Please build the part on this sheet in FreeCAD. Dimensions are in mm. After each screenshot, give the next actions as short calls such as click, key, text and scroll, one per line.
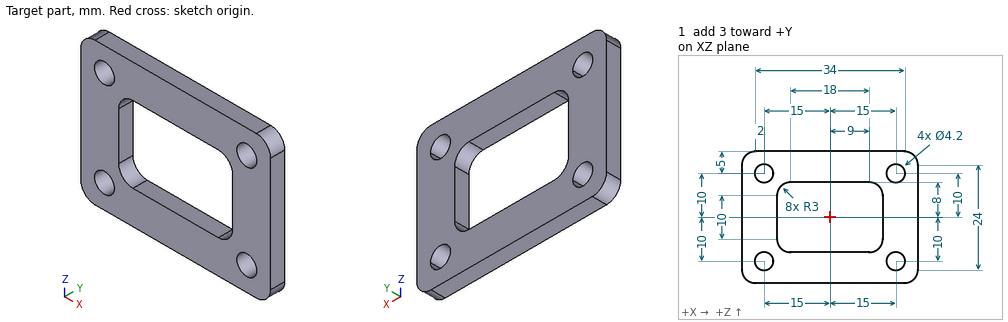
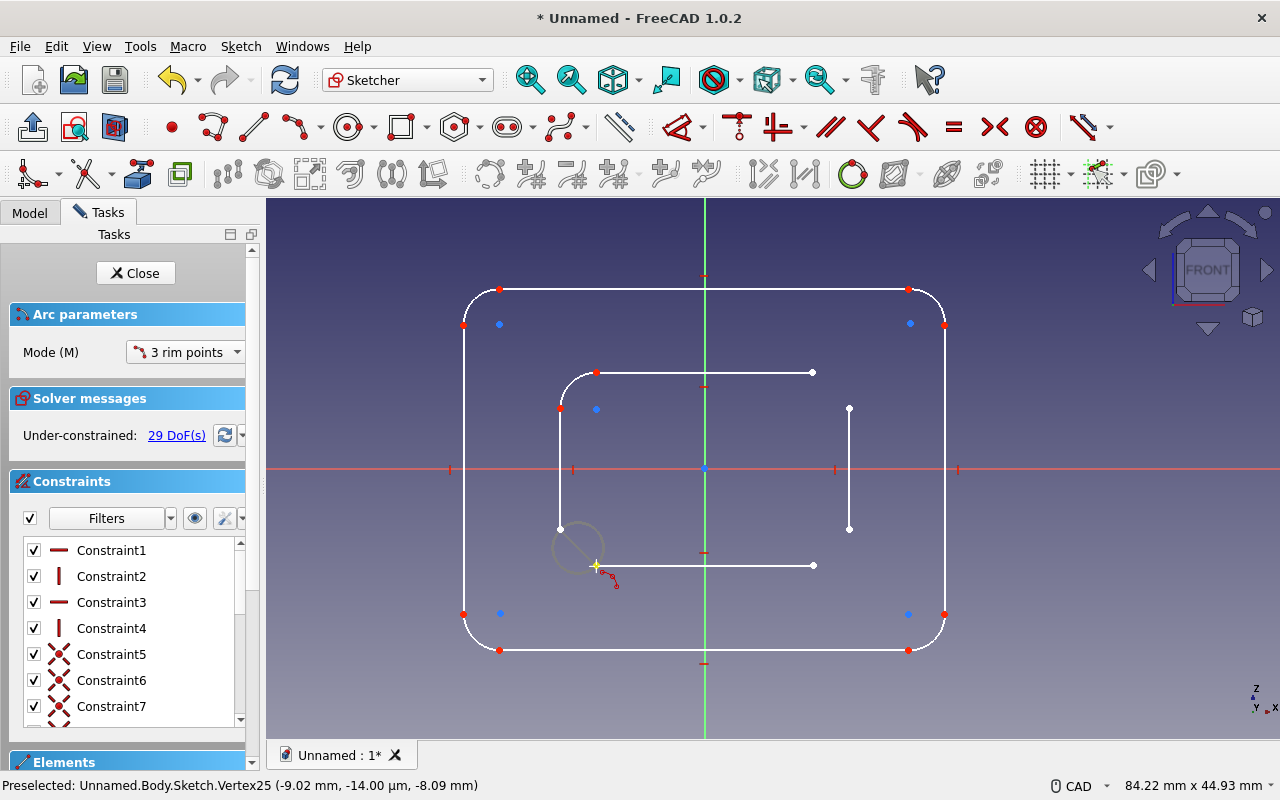
scroll(571, 554, up, 3)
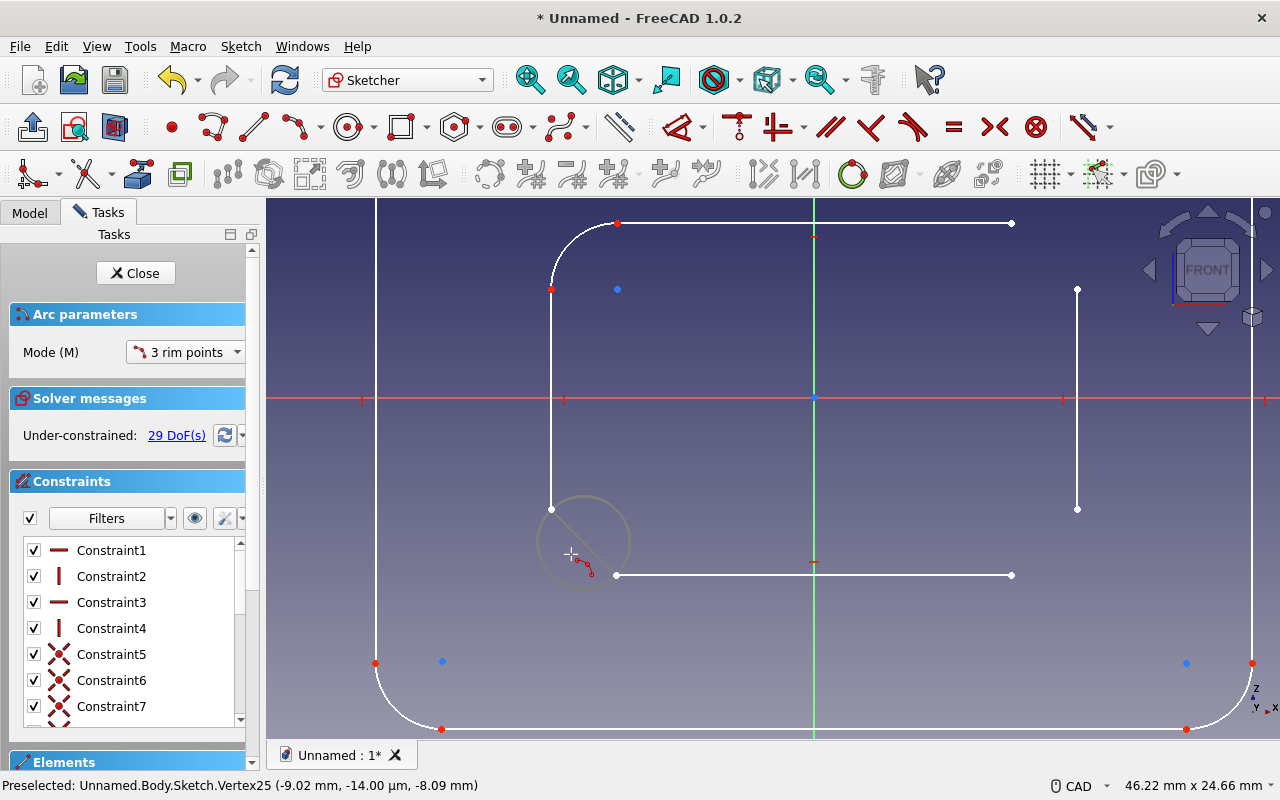
click(570, 554)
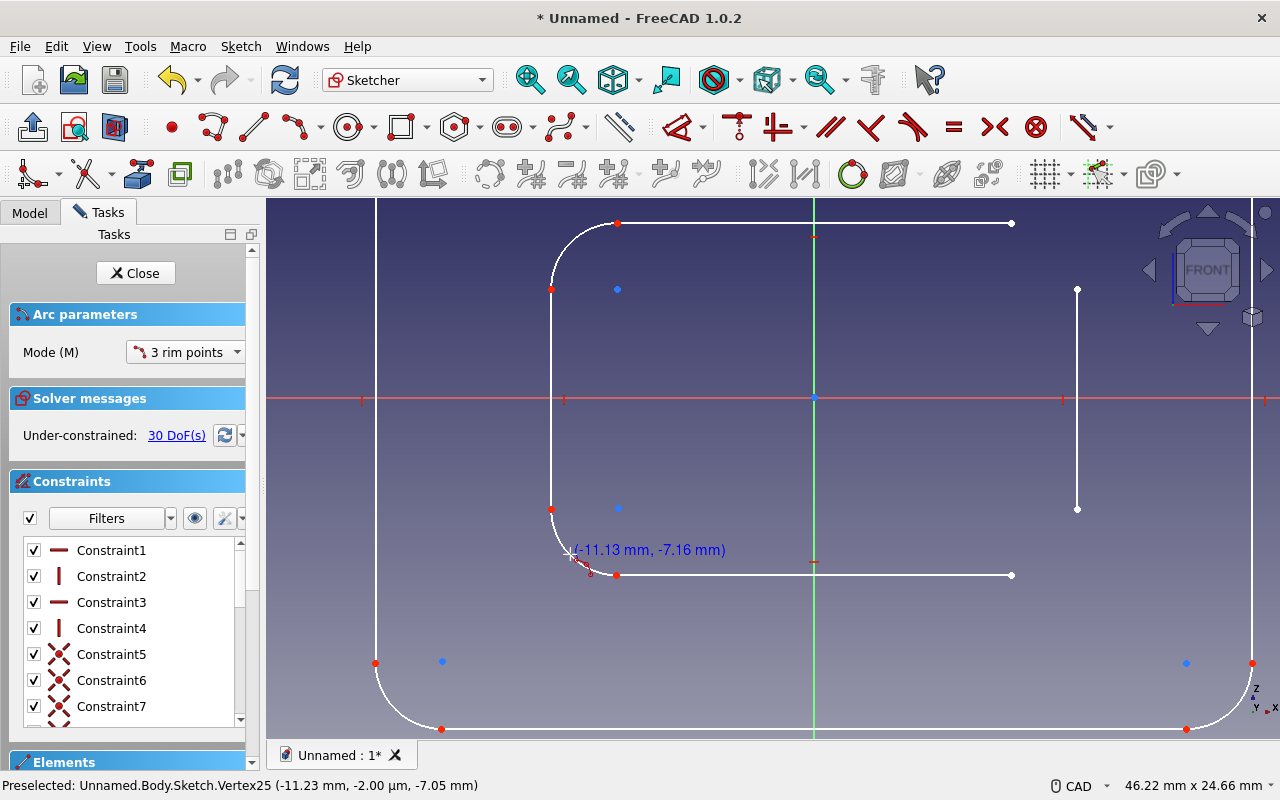
click(1012, 575)
click(1077, 510)
click(1058, 554)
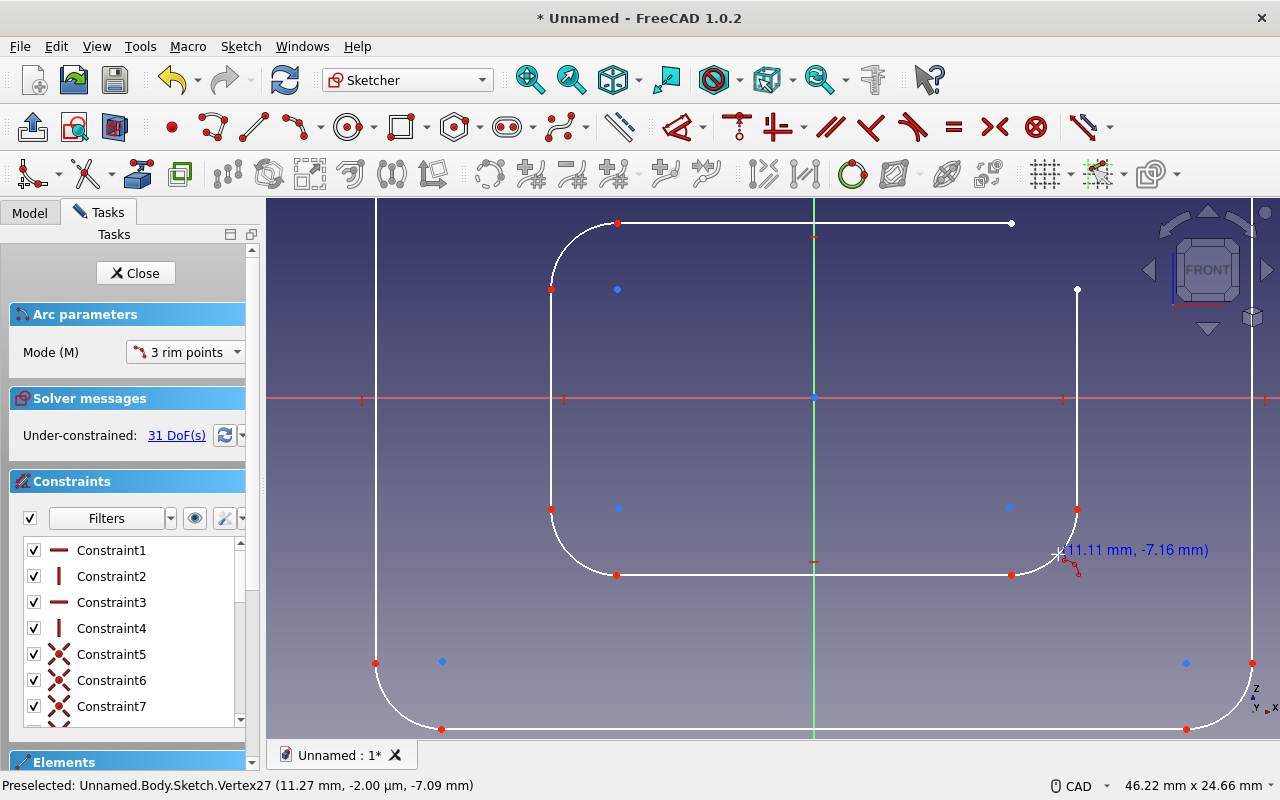
click(1077, 289)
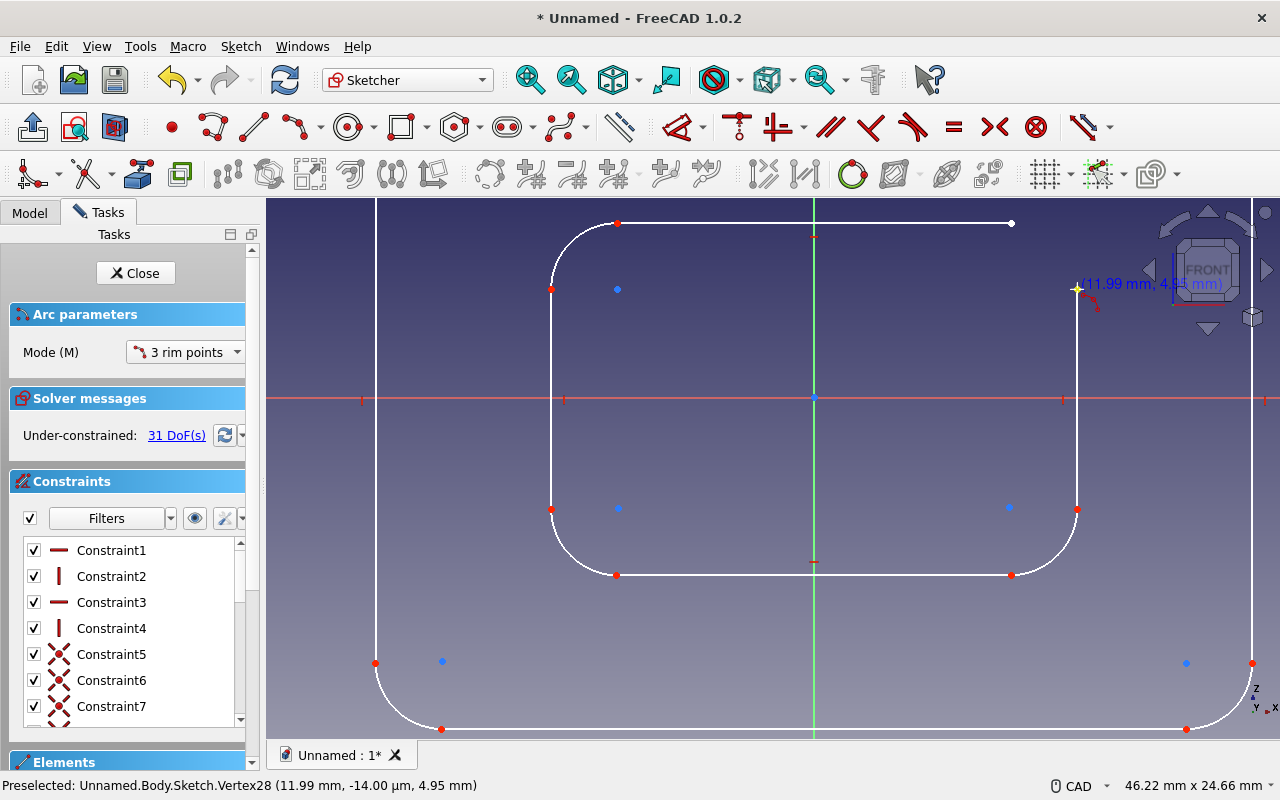
scroll(571, 554, down, 3)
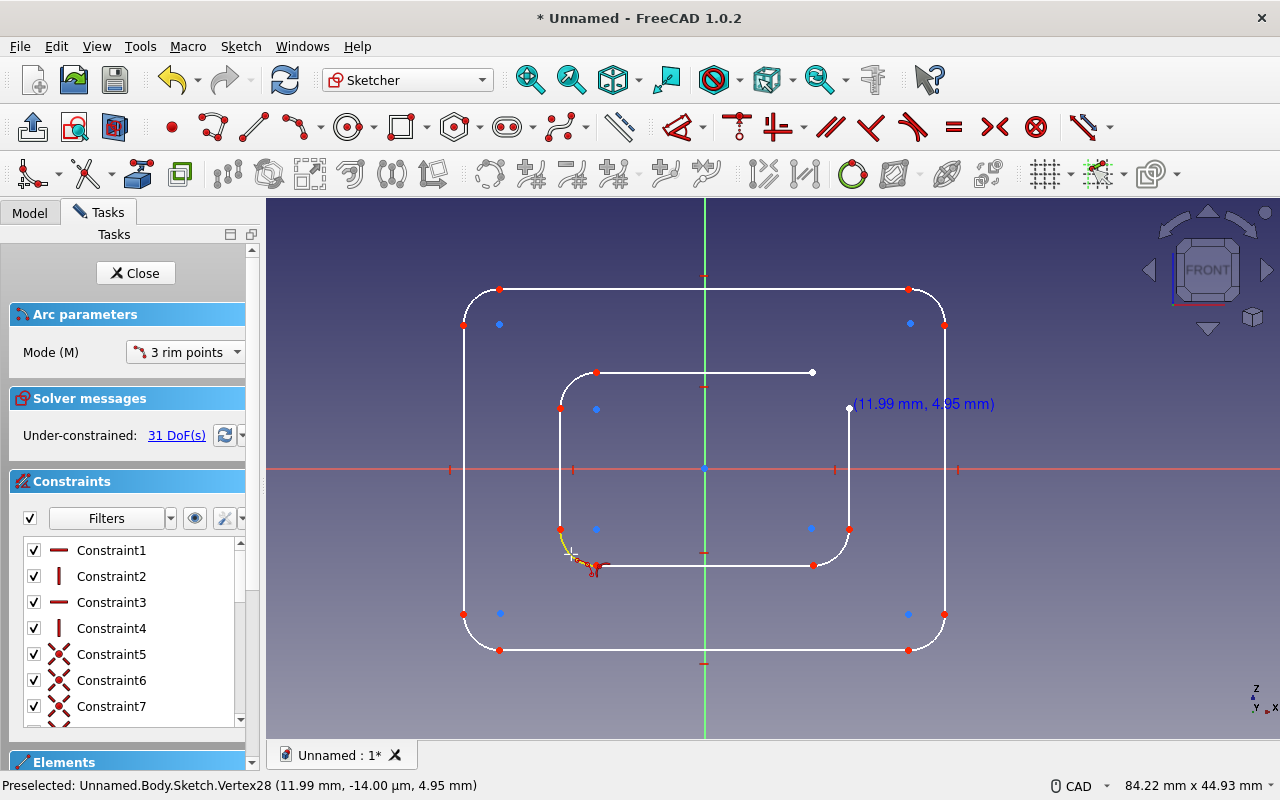
click(813, 373)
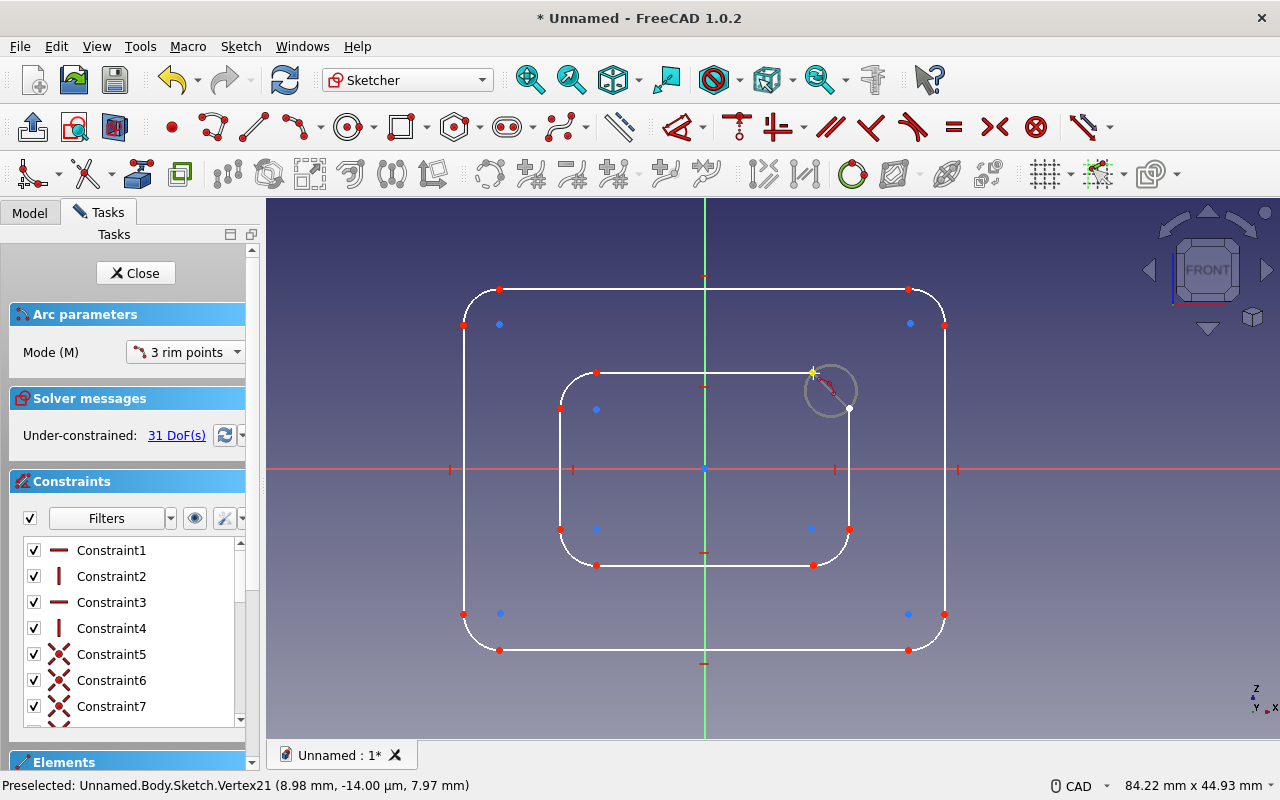
scroll(838, 383, up, 3)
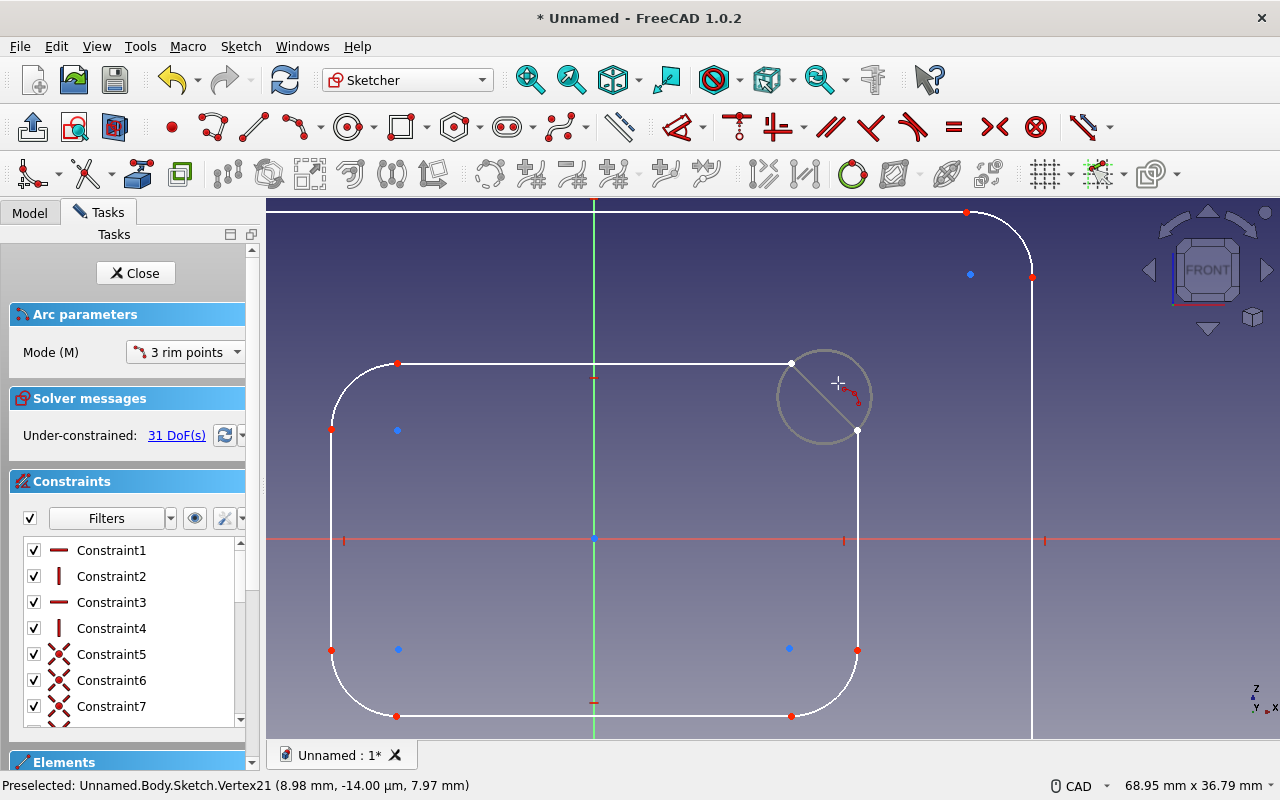
click(838, 383)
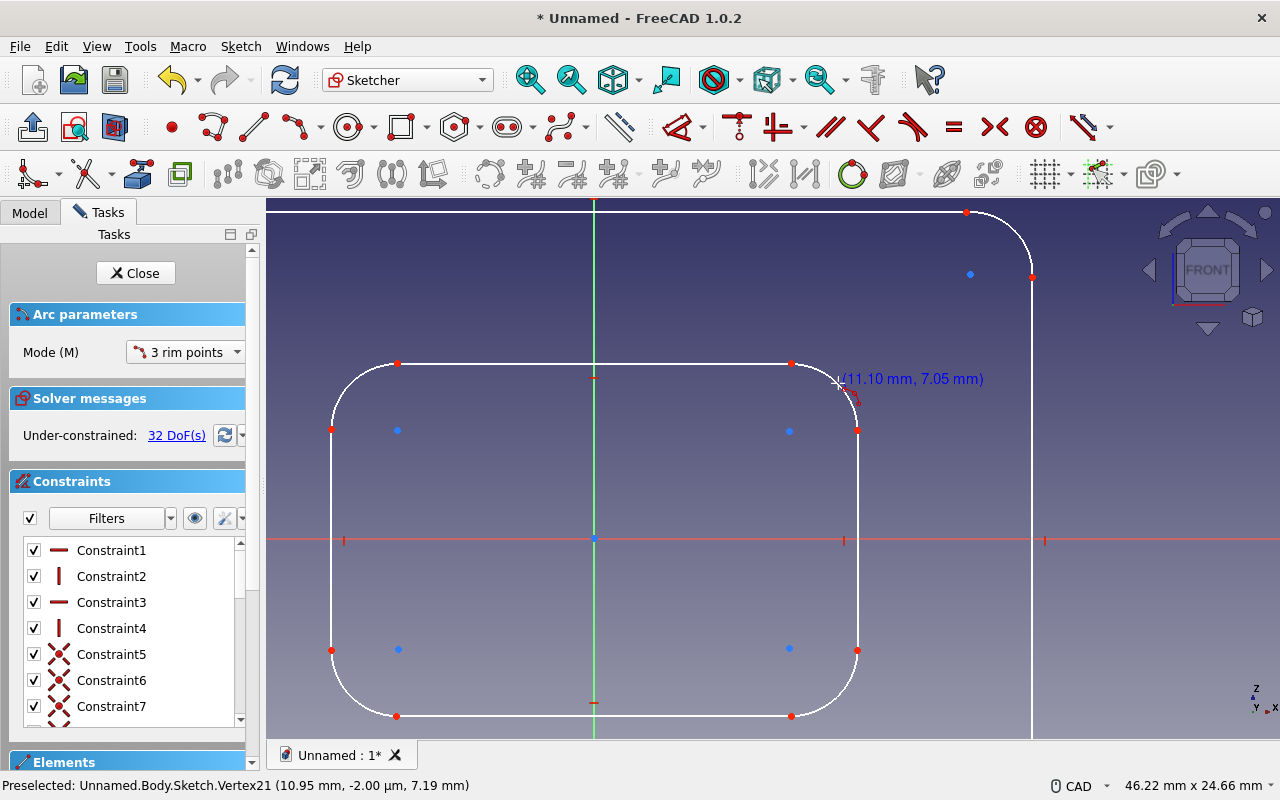
click(348, 128)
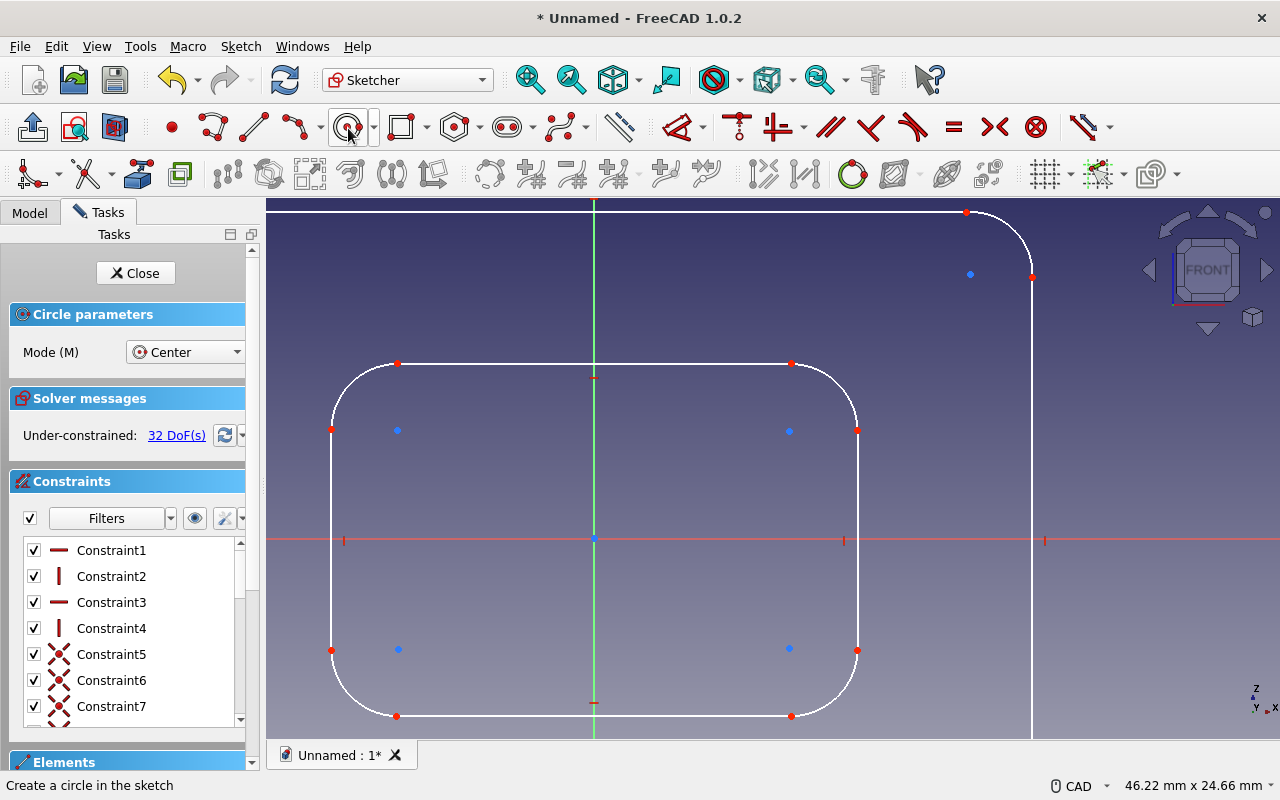
scroll(838, 383, down, 3)